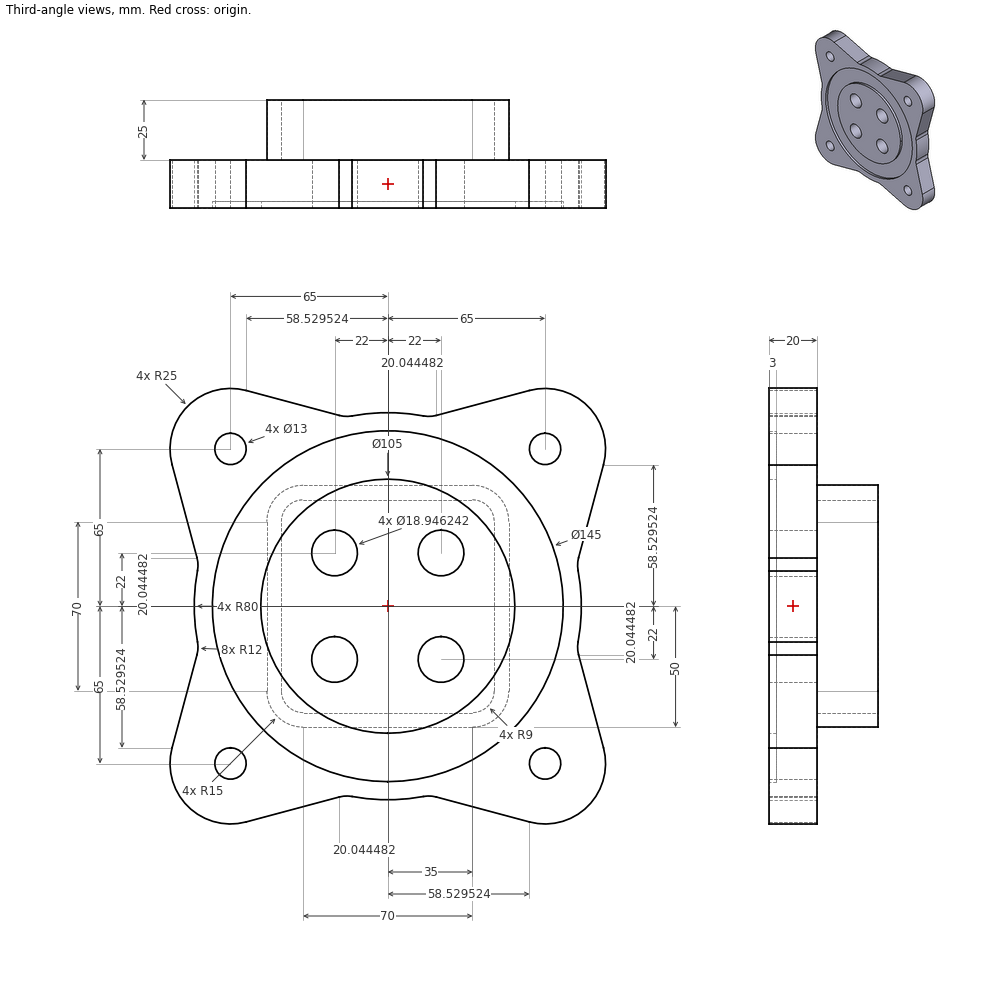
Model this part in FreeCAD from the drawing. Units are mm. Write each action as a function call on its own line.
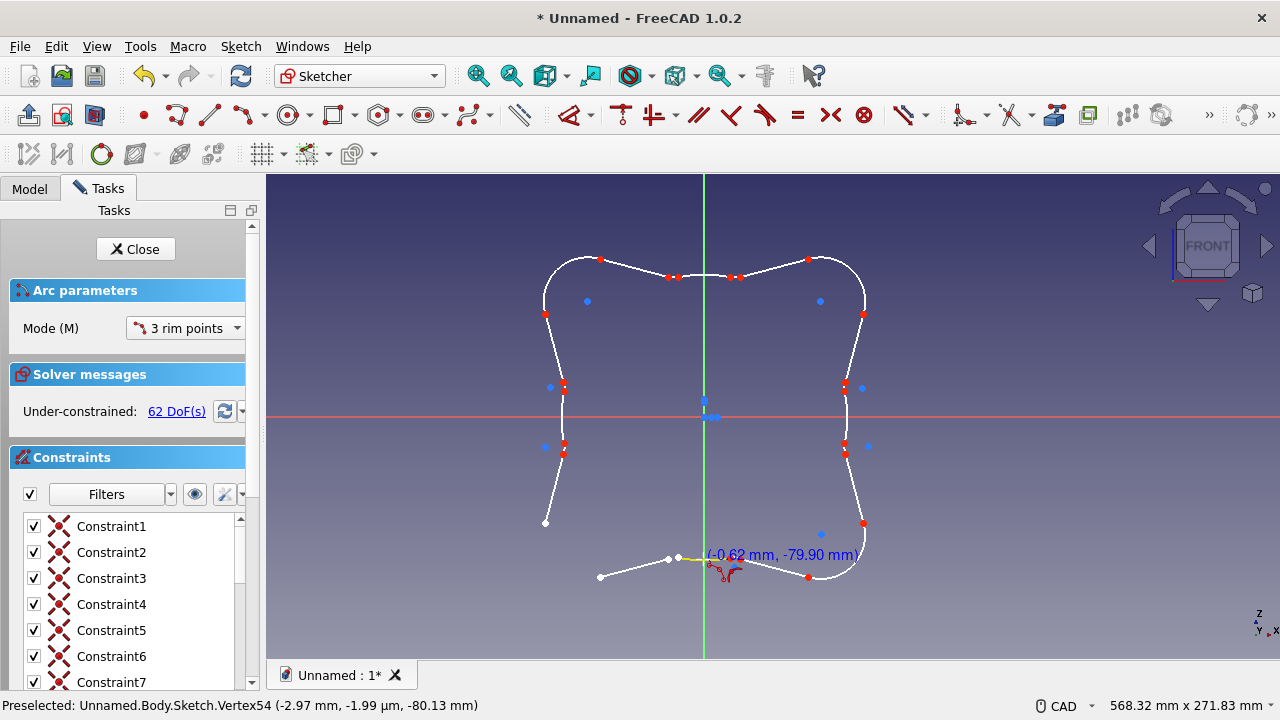
scroll(678, 558, up, 3)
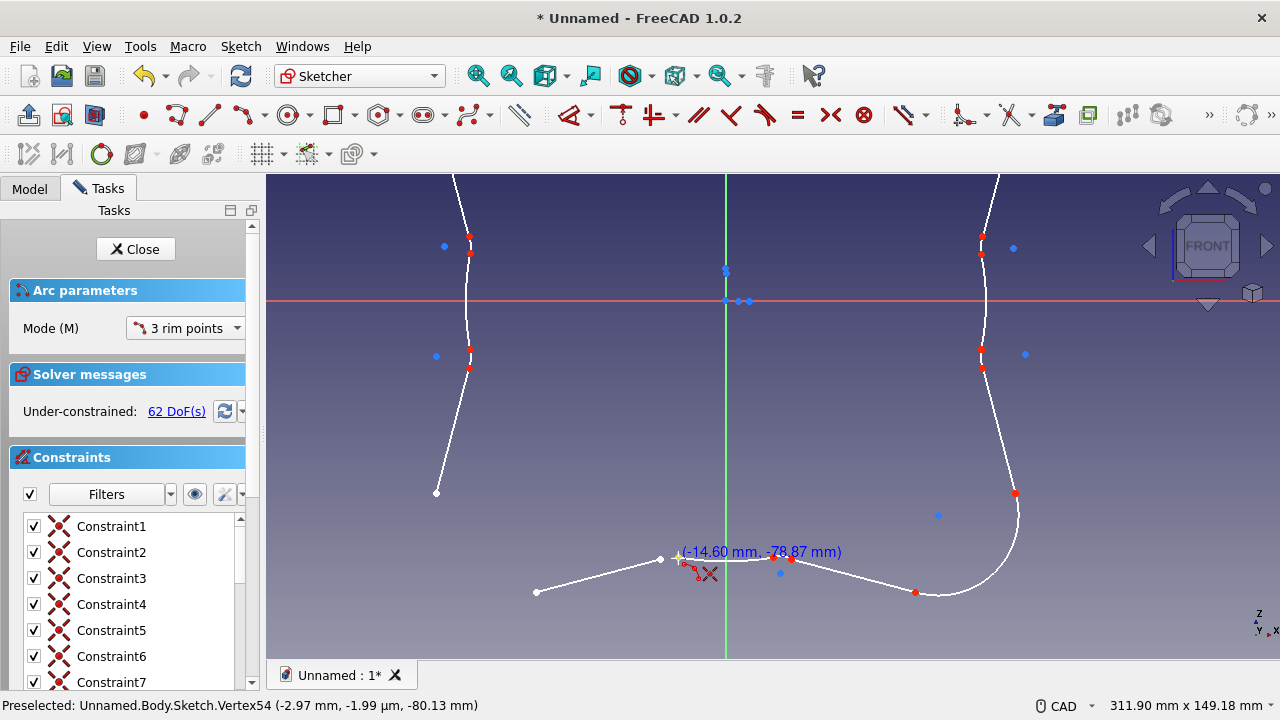
click(678, 557)
click(660, 559)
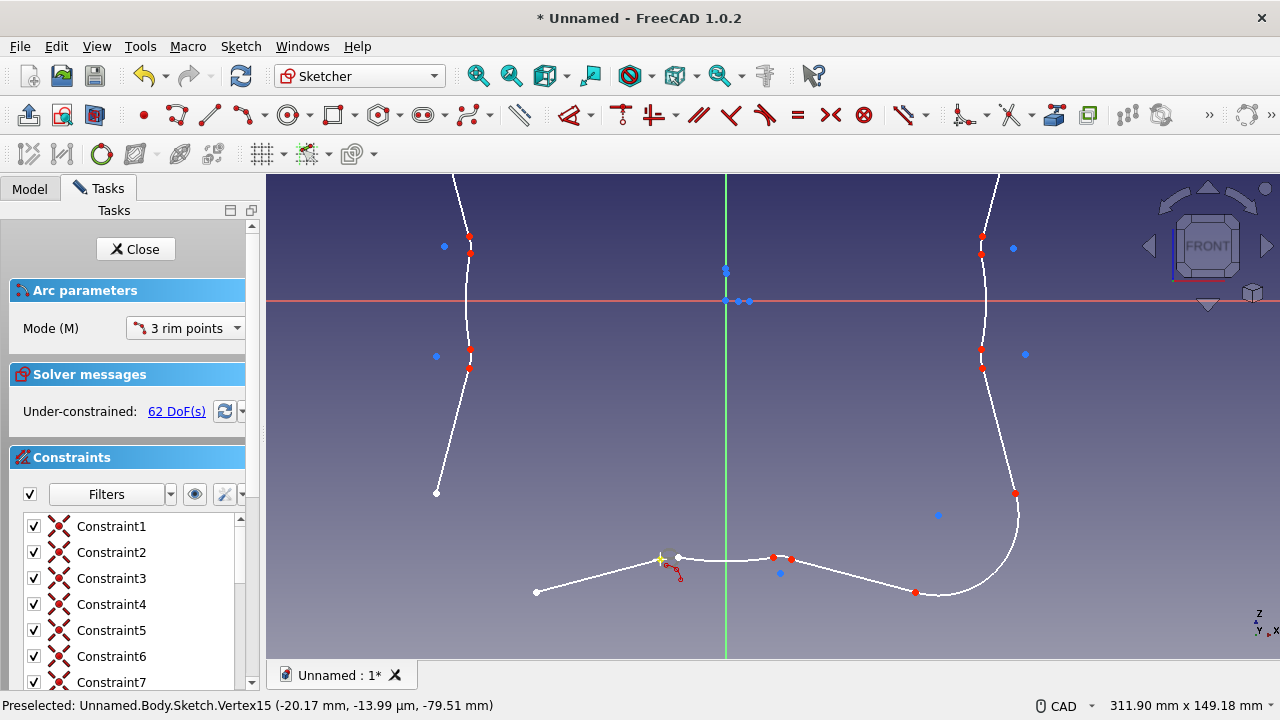
scroll(669, 556, up, 14)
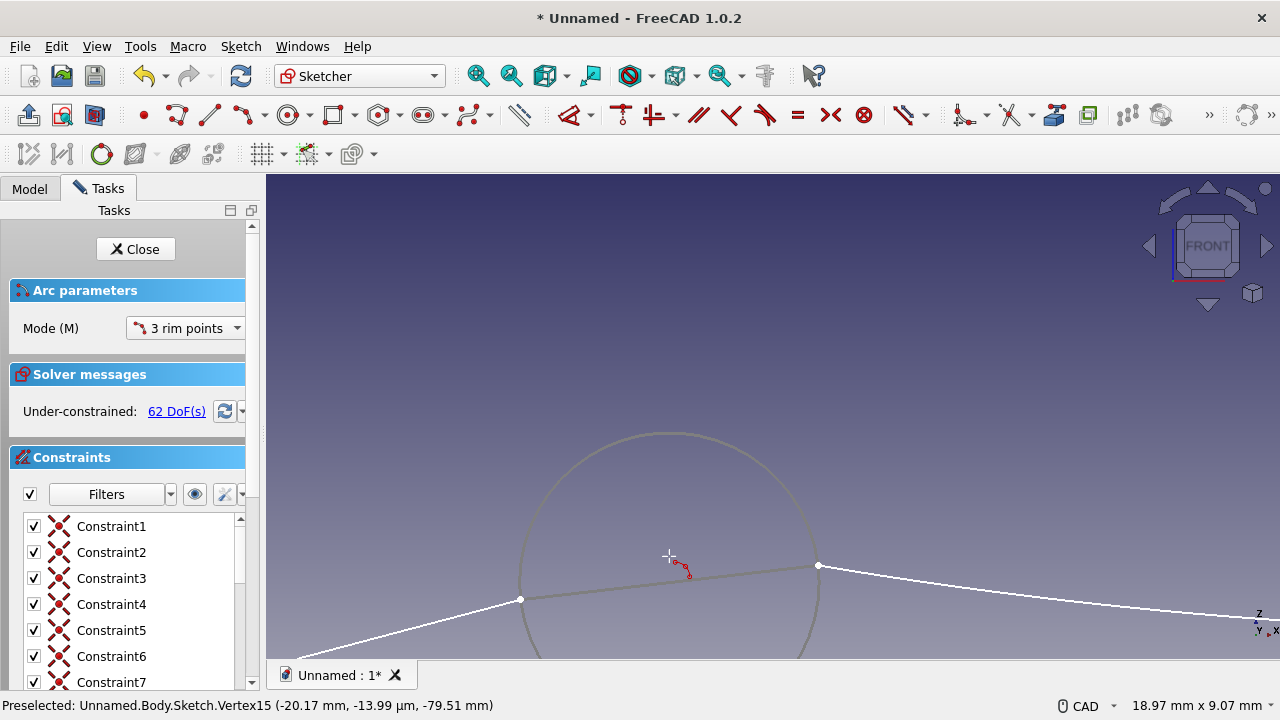
click(669, 542)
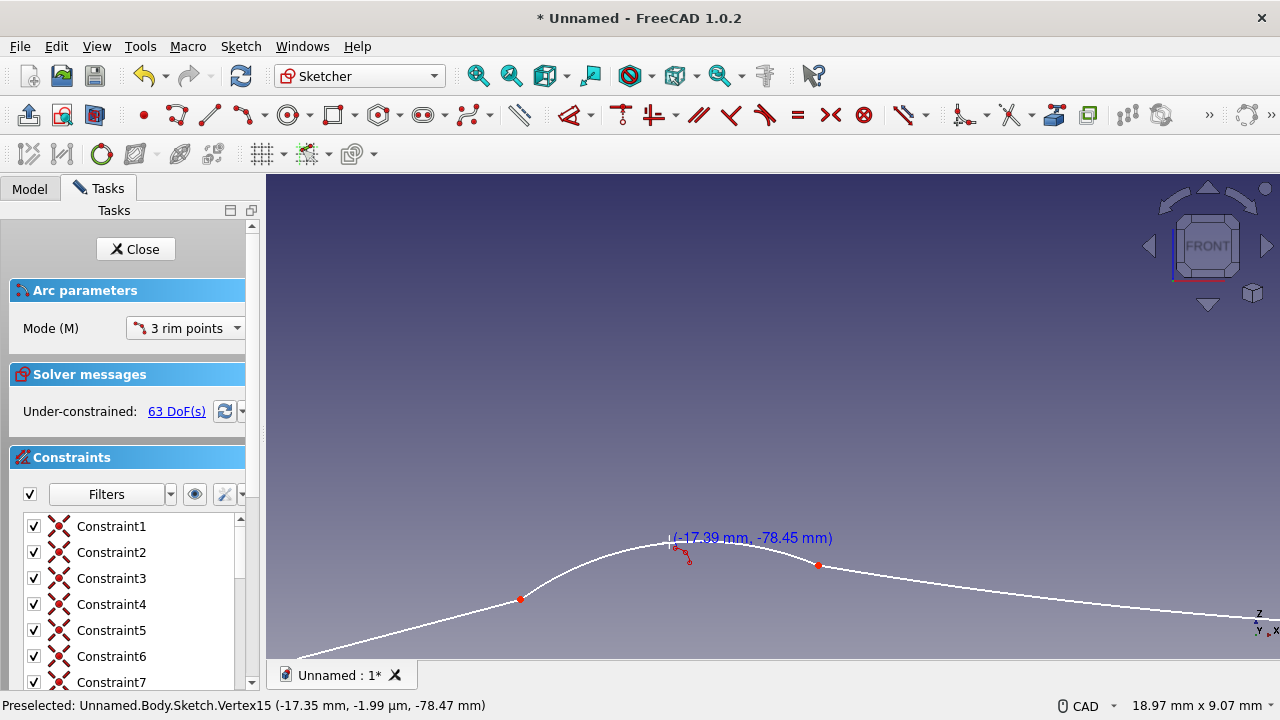
scroll(674, 557, down, 17)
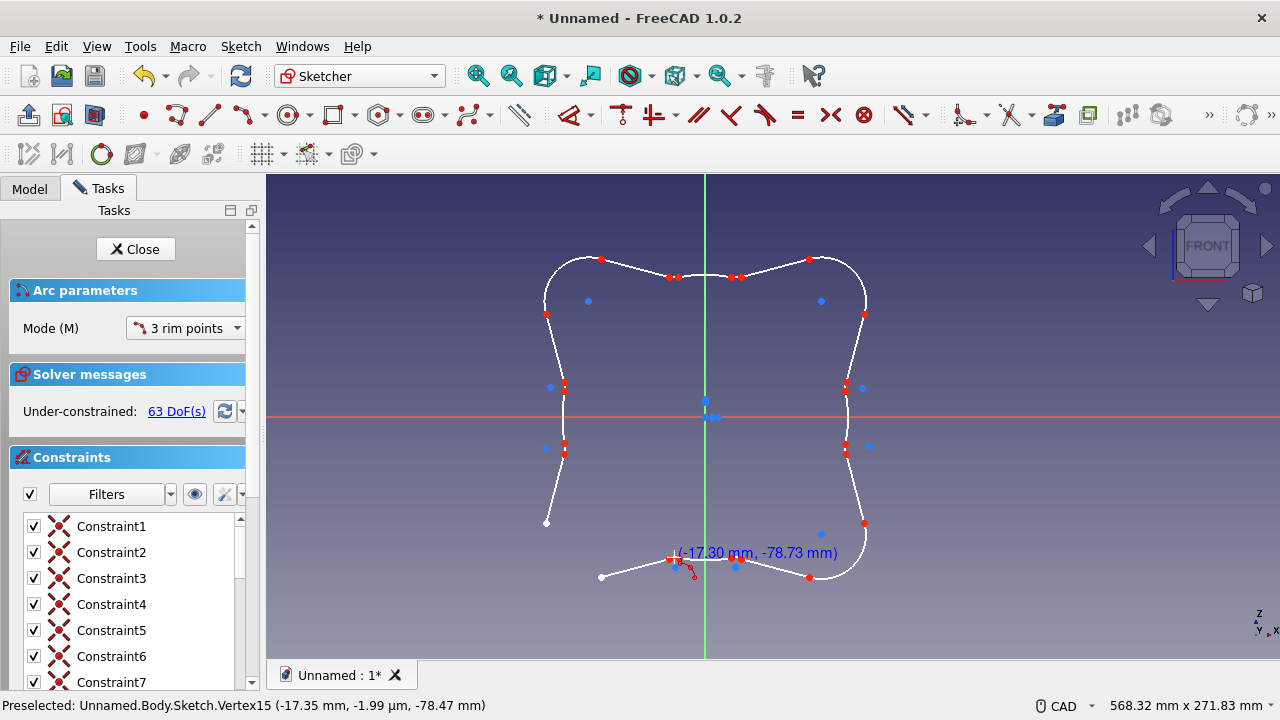
click(601, 577)
click(546, 523)
click(558, 565)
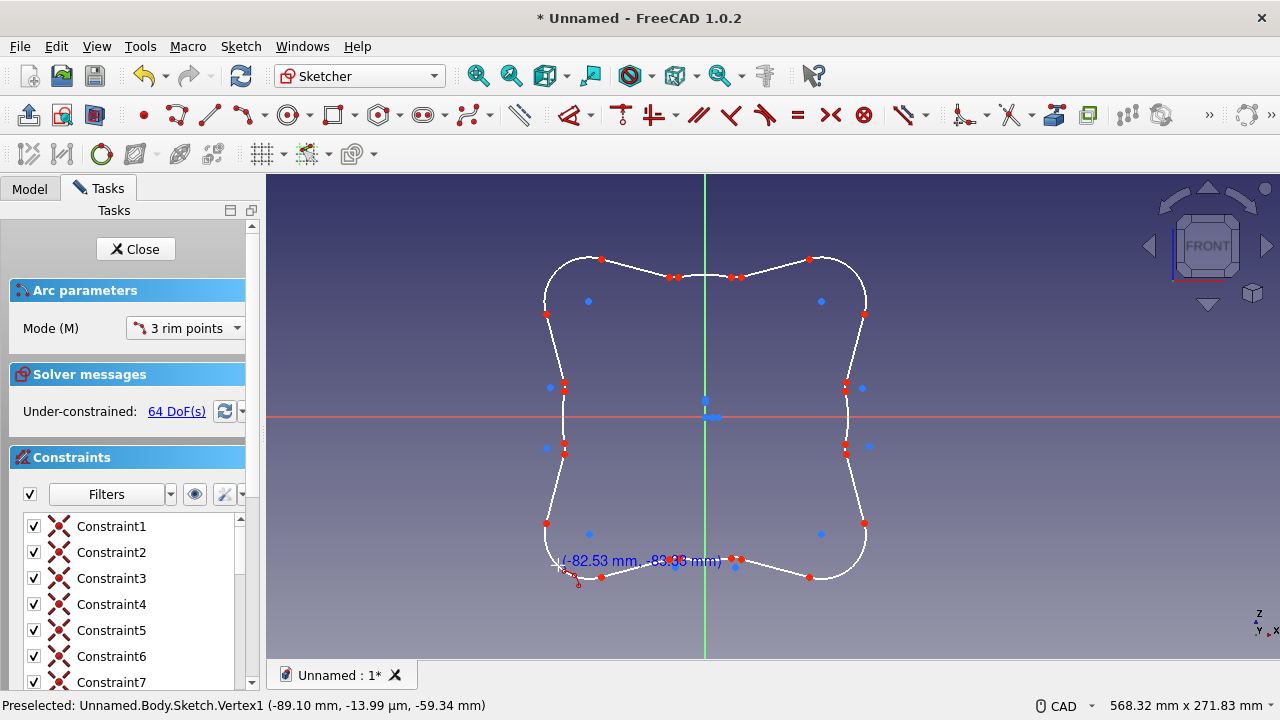
click(288, 116)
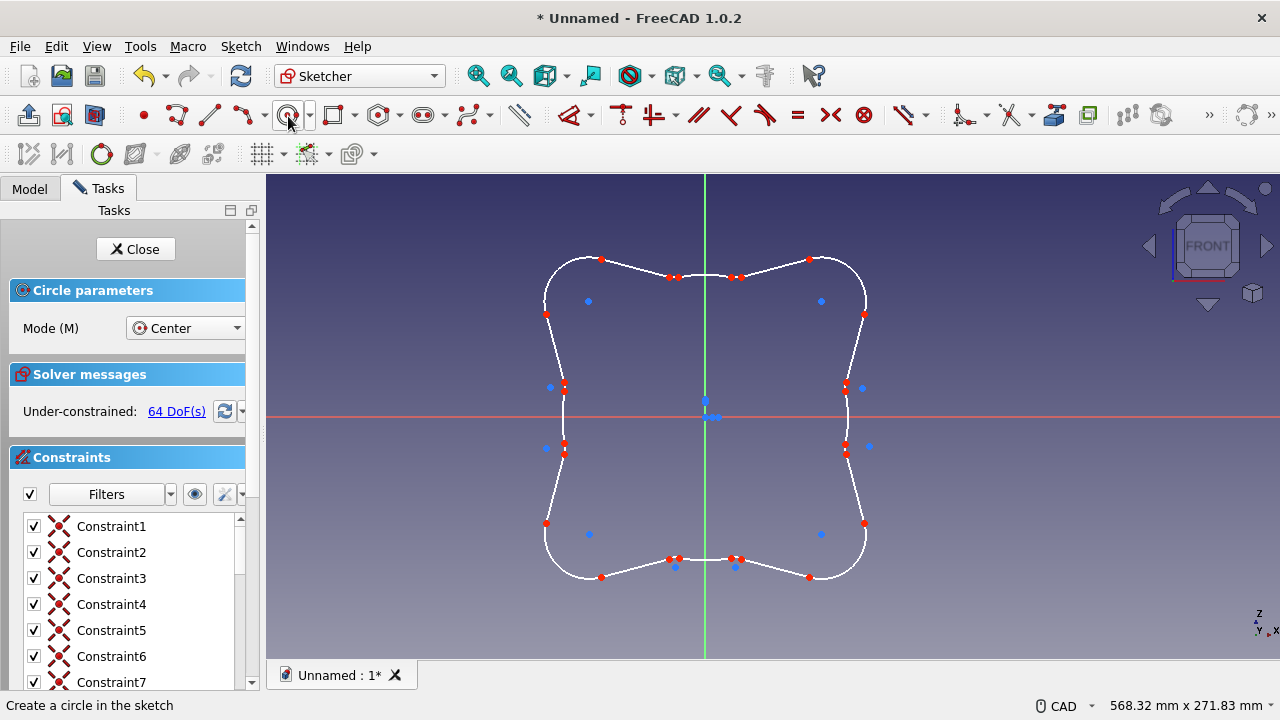
scroll(589, 301, up, 4)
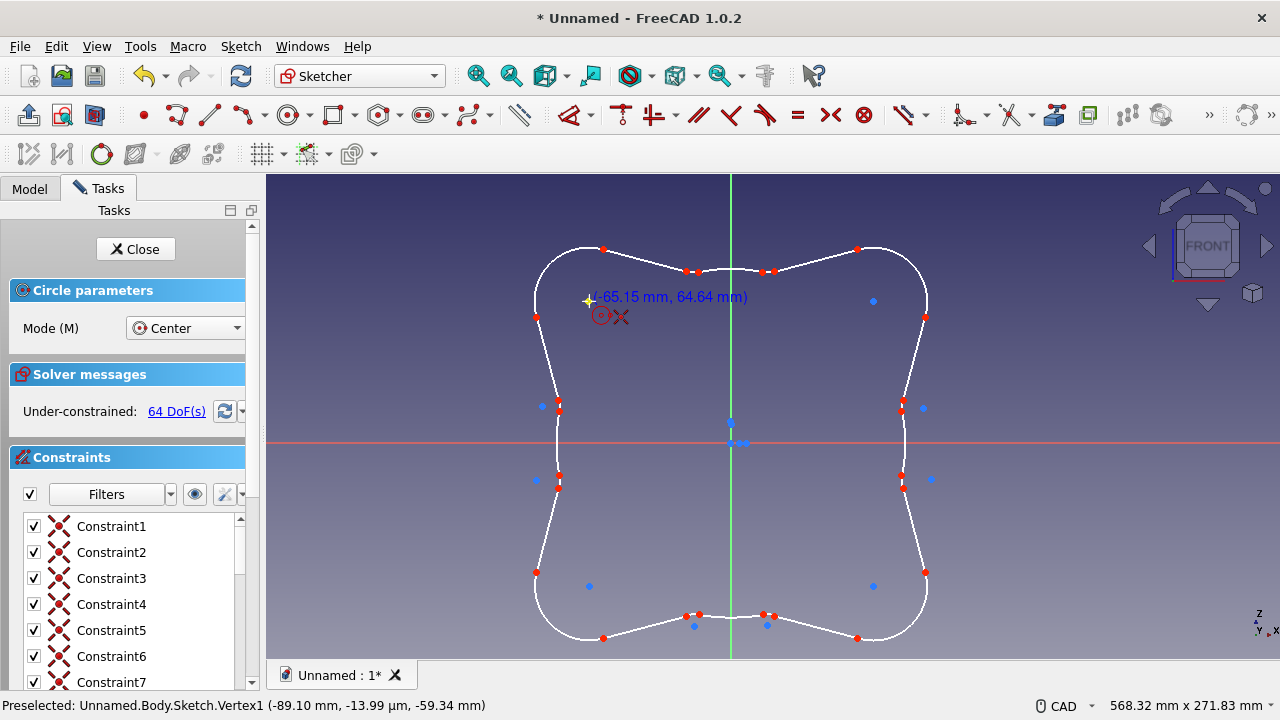
click(589, 301)
move(607, 283)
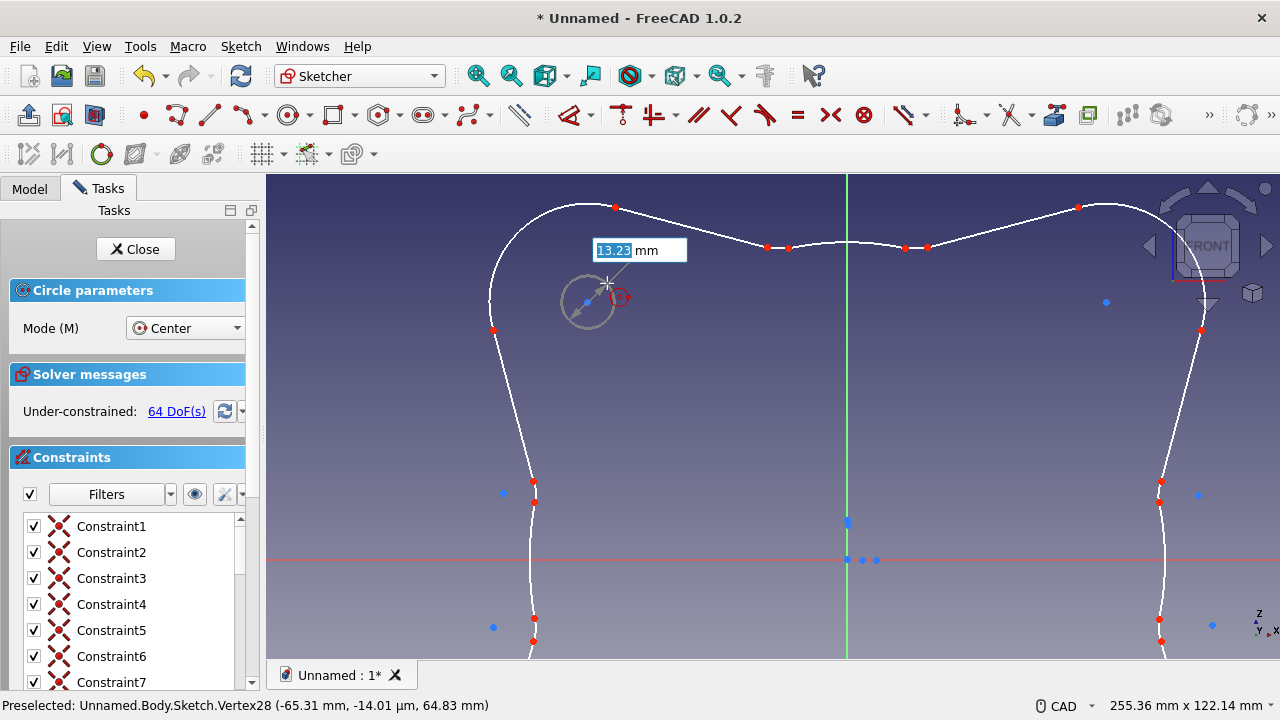
text(13)
key(Return)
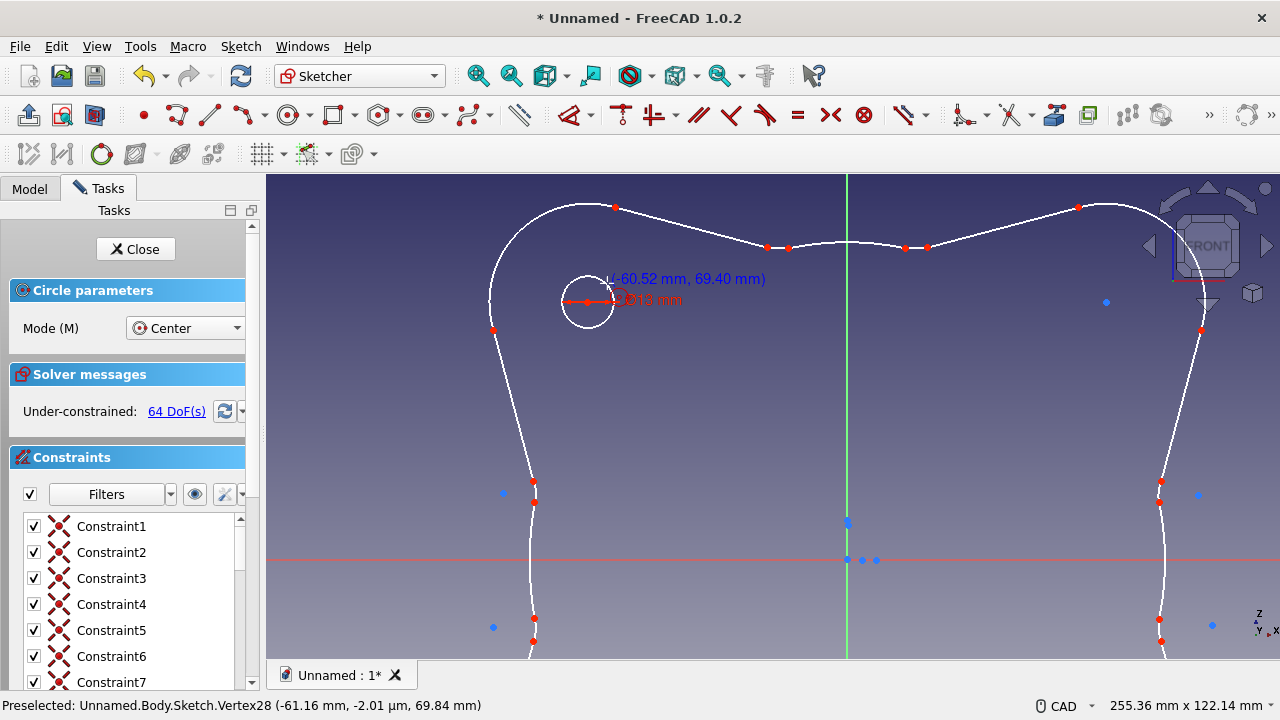
click(1105, 301)